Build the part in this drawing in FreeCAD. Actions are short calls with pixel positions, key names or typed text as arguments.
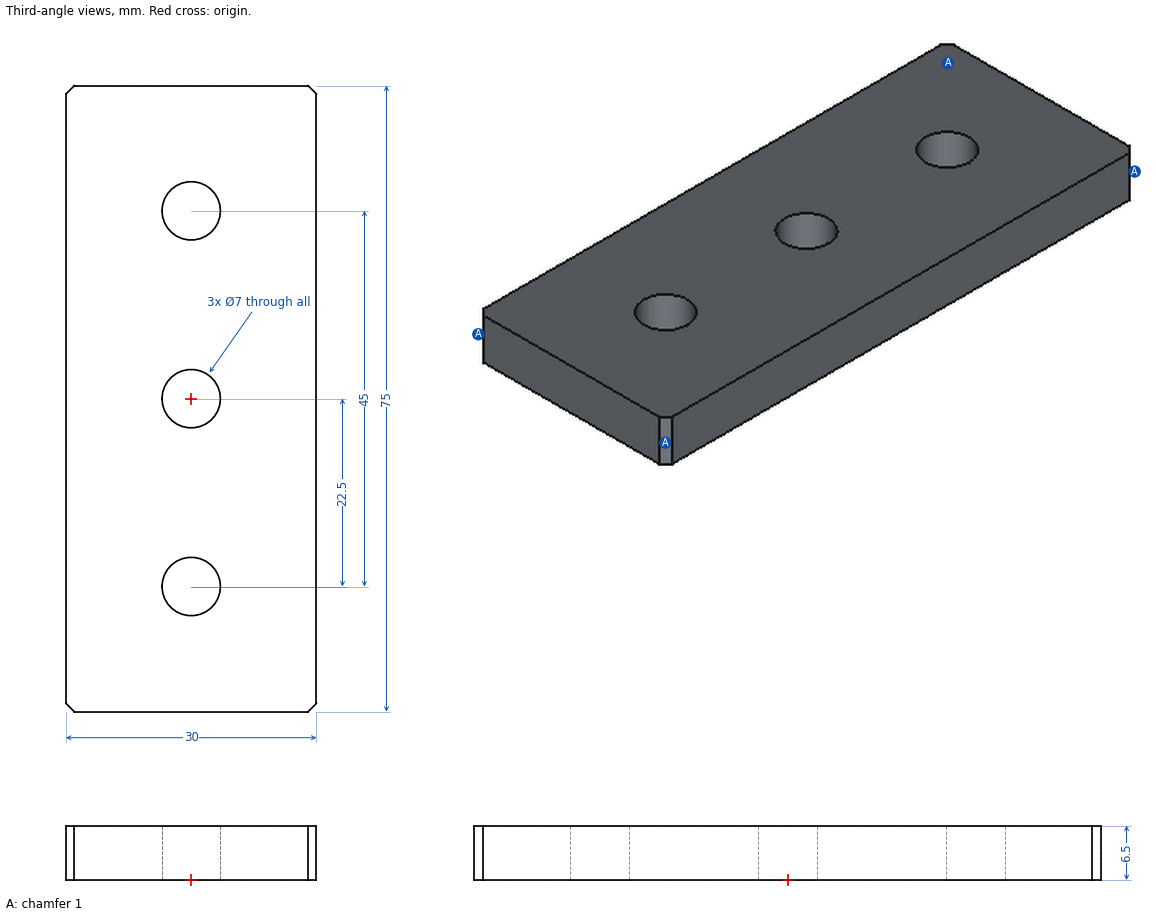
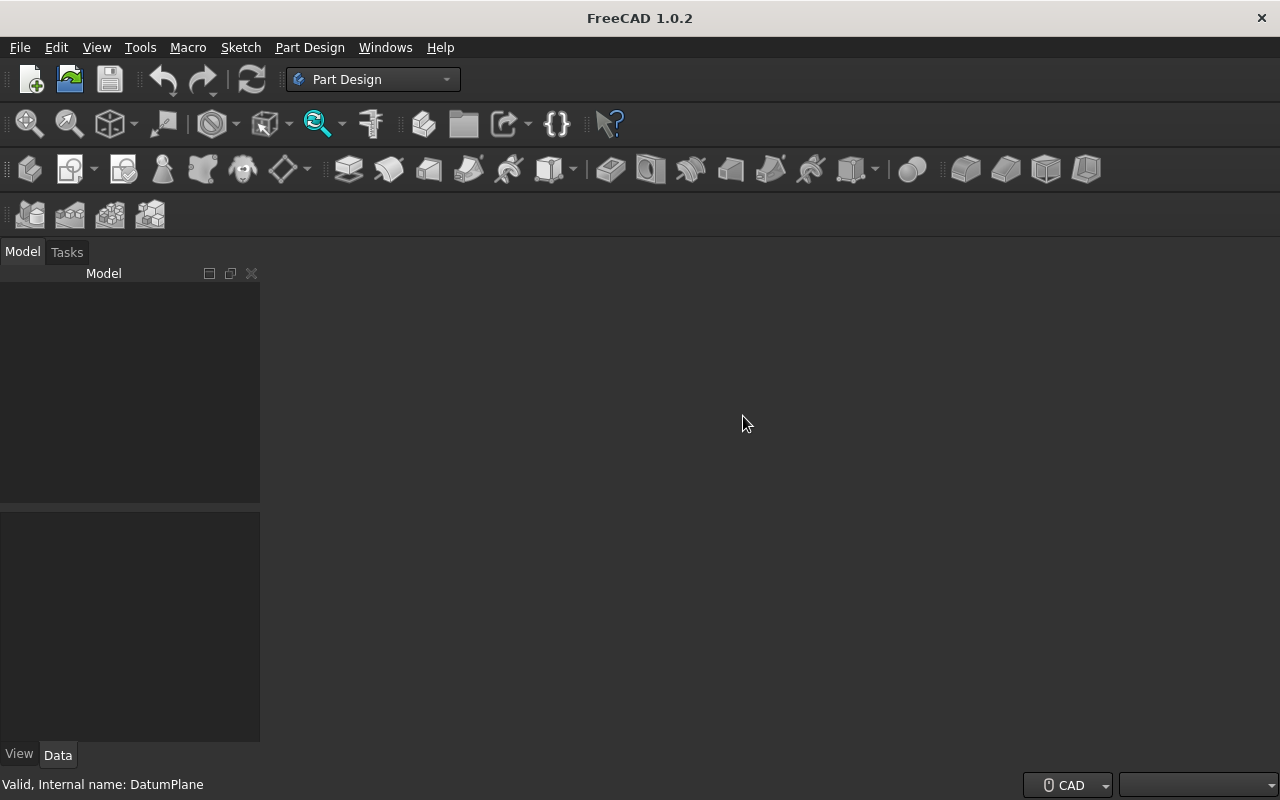
key(ctrl+n)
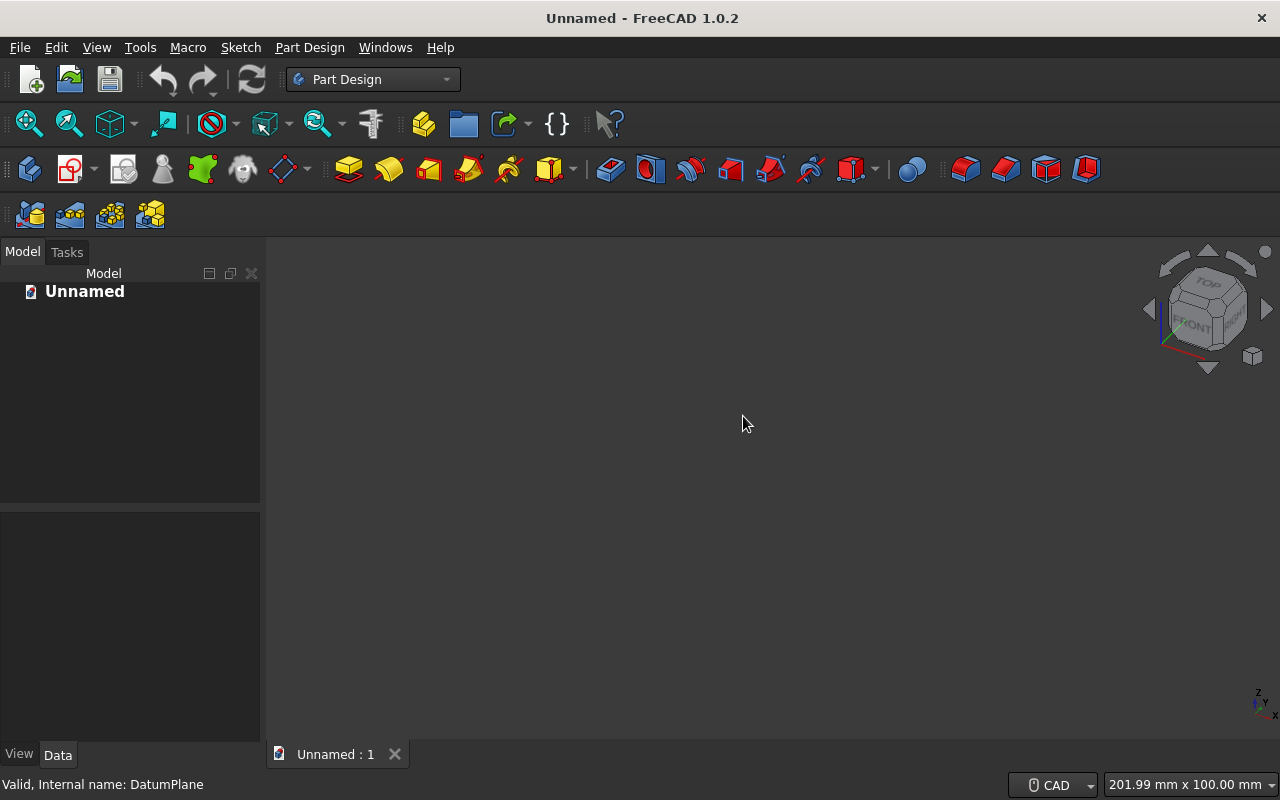
click(70, 170)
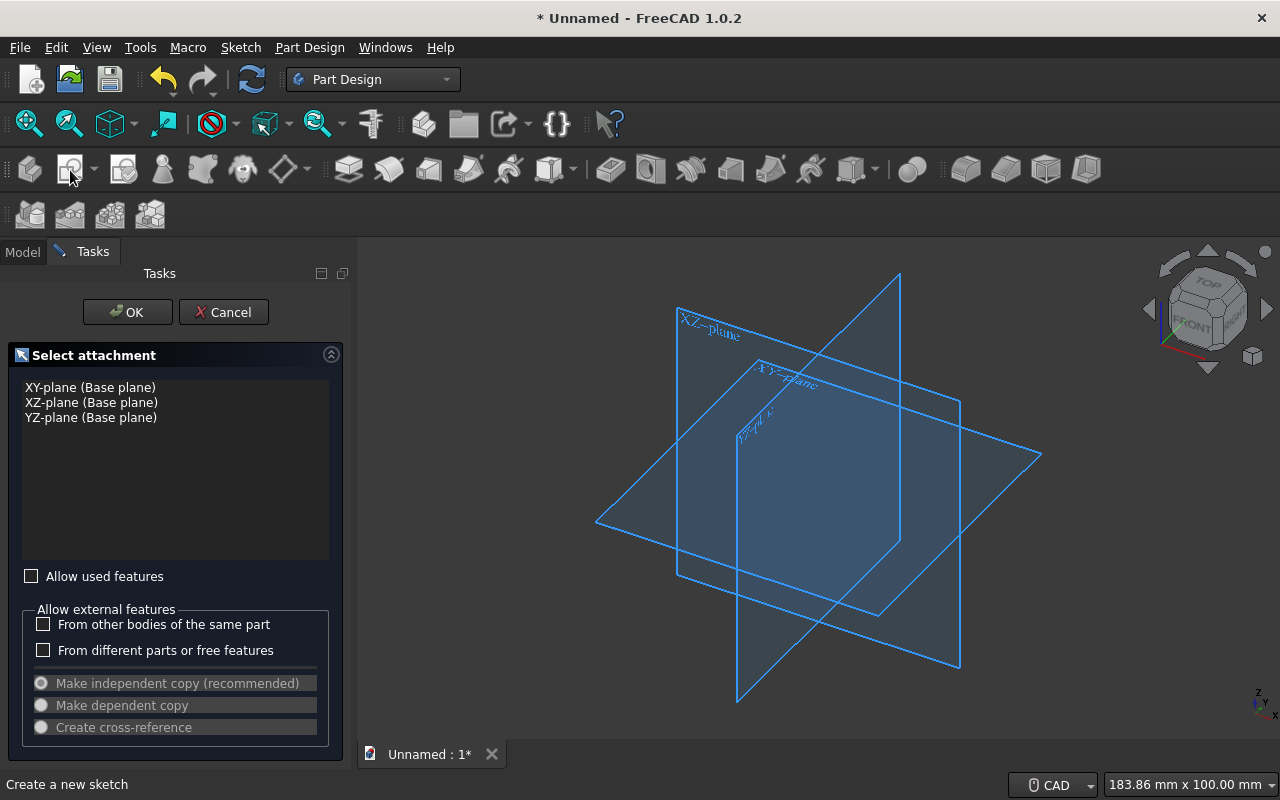
click(82, 388)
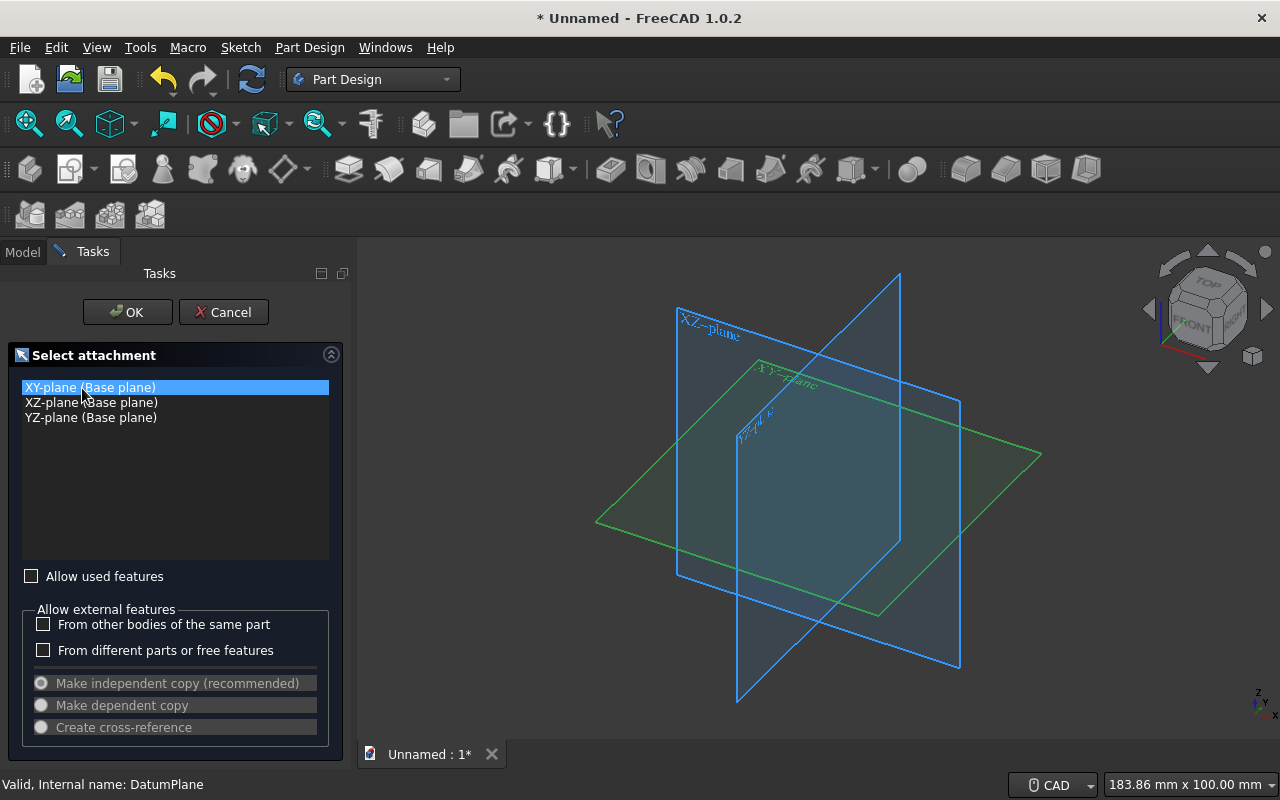
click(128, 312)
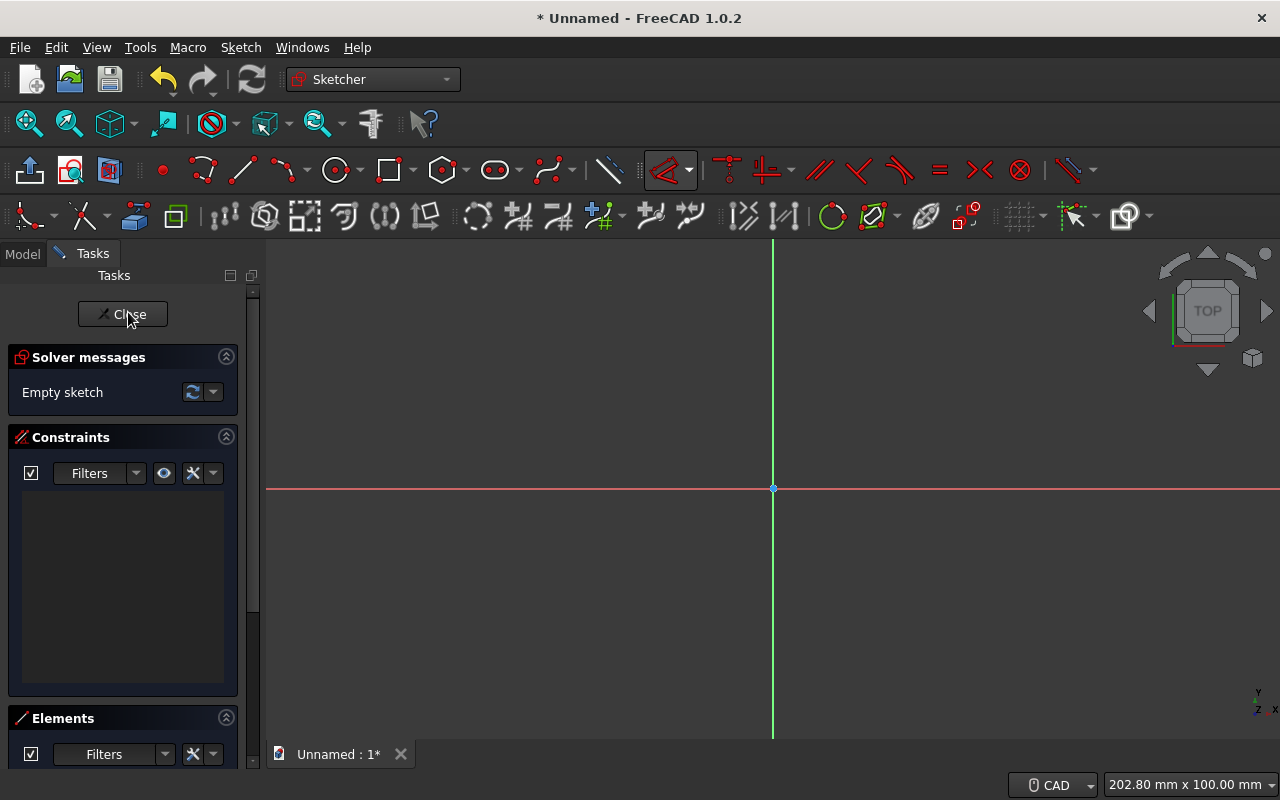
key(g)
key(v)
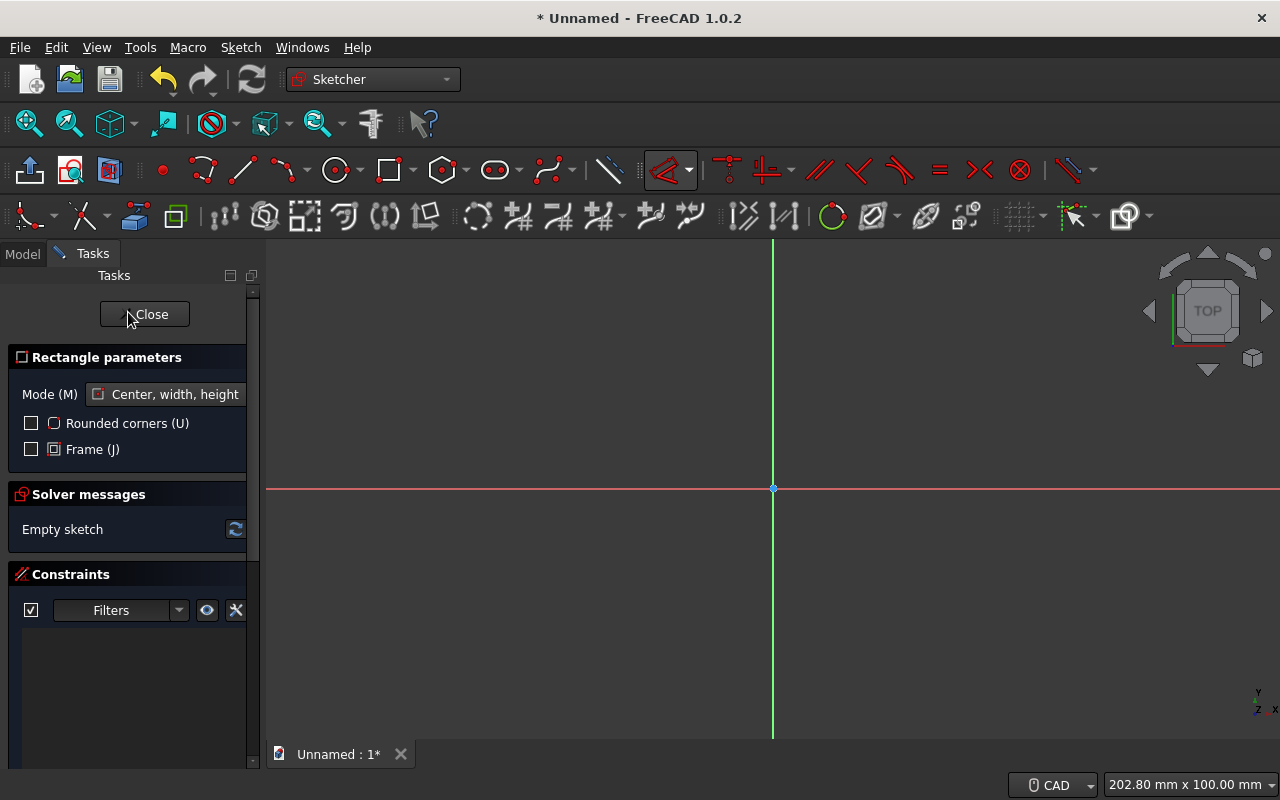
click(773, 489)
click(848, 302)
key(Escape)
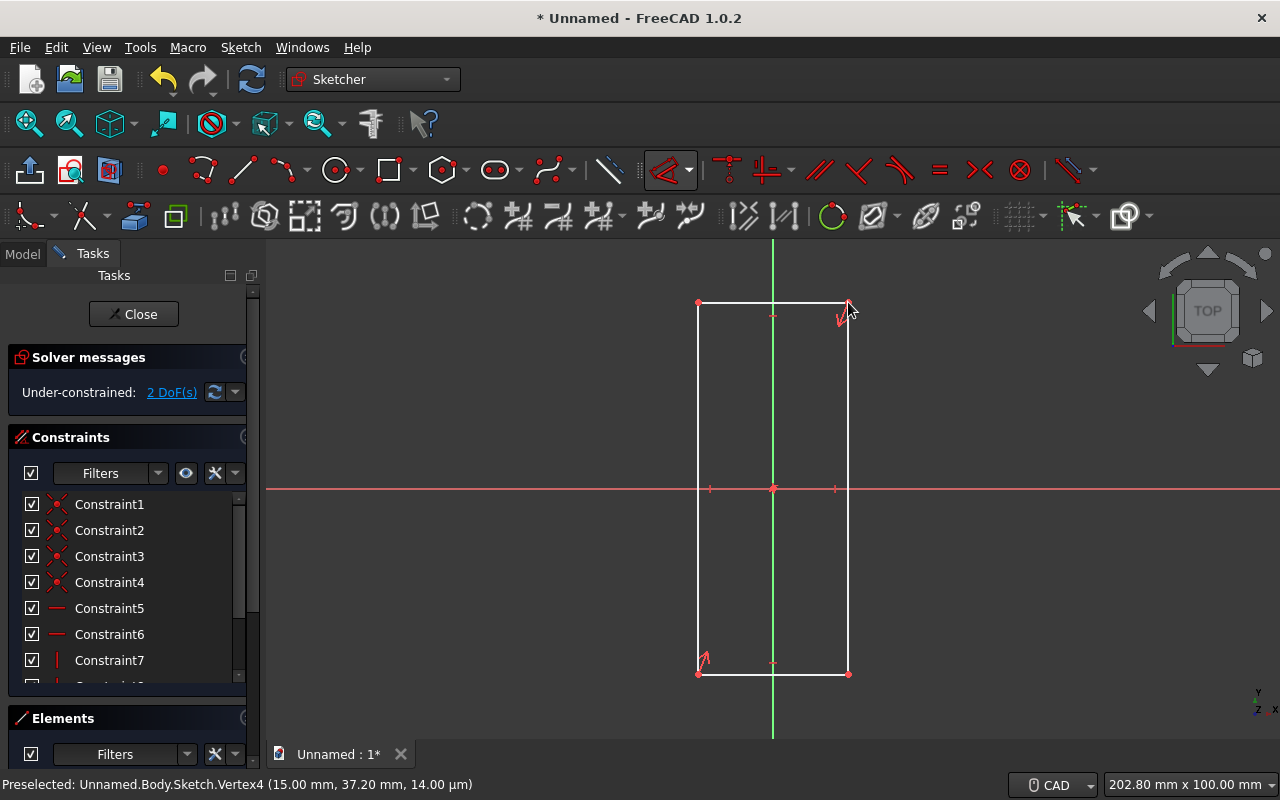
key(d)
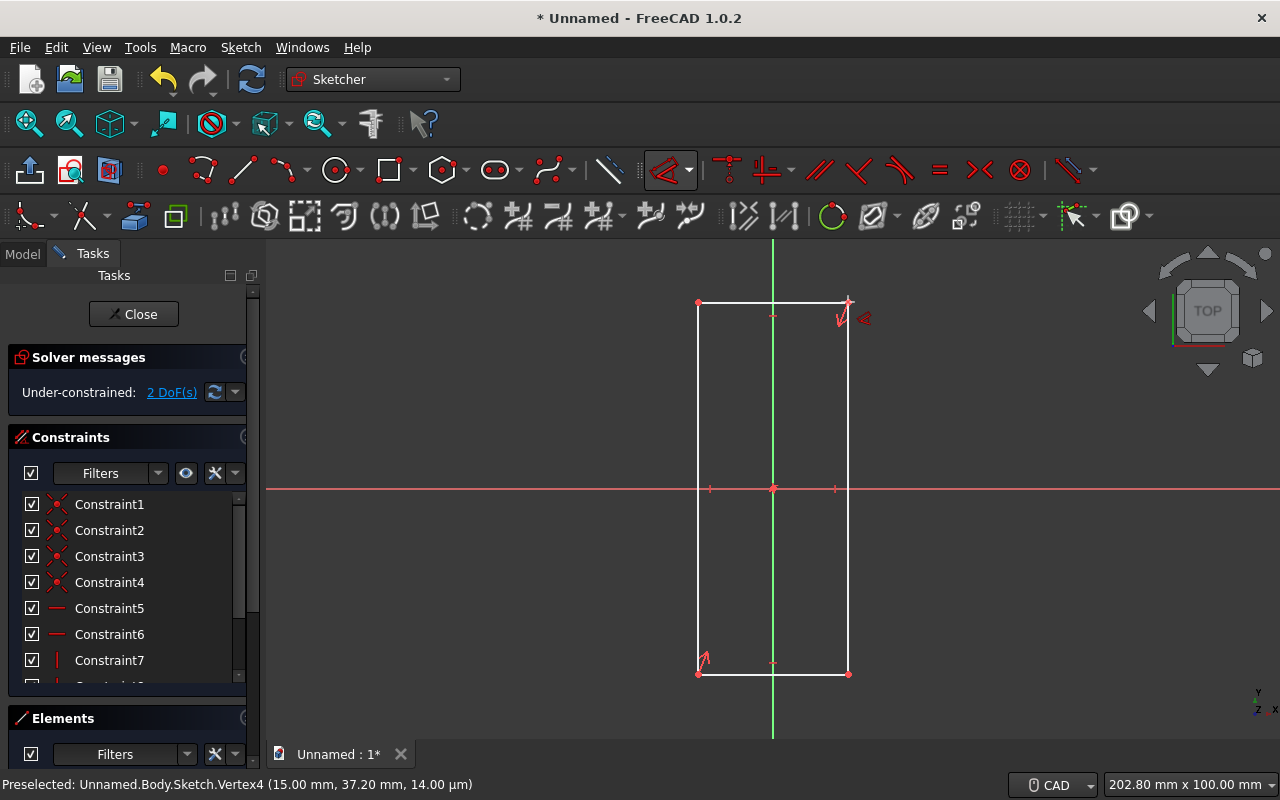
click(743, 675)
click(739, 709)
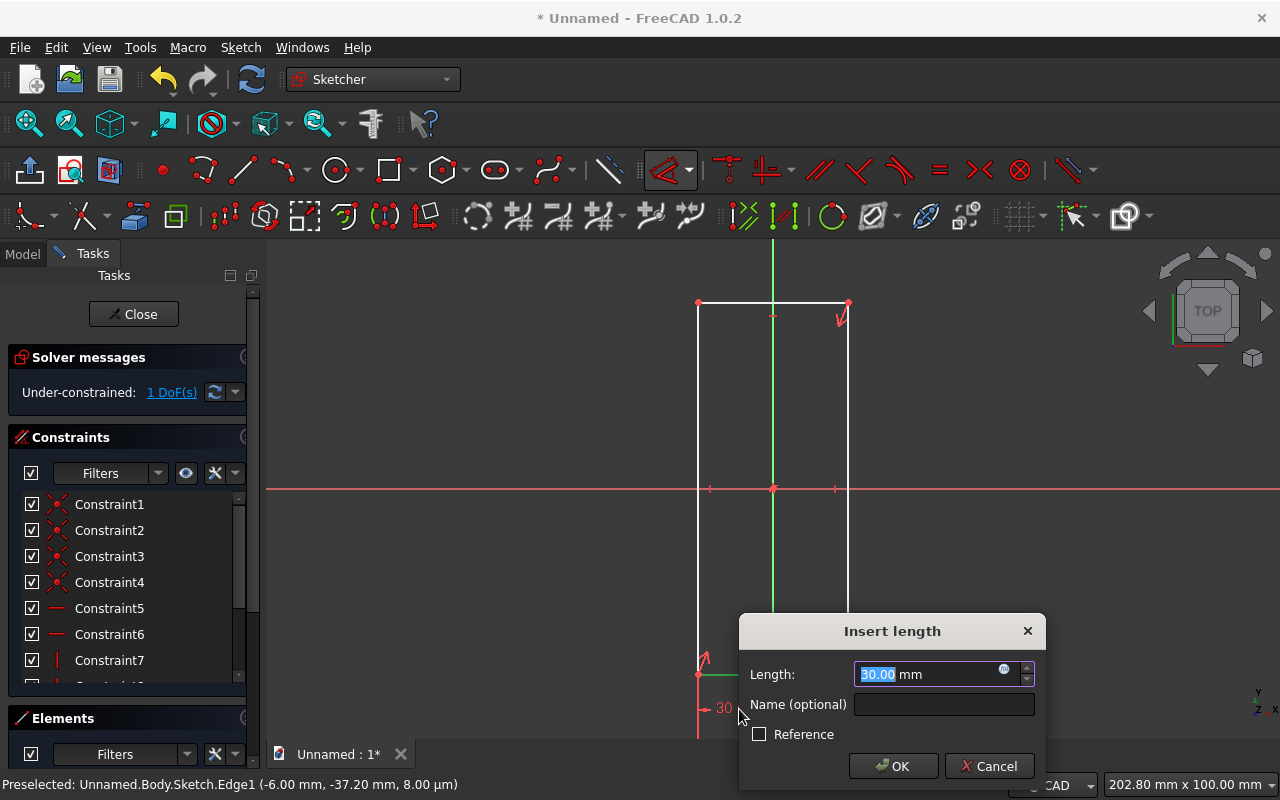
text(30)
key(Return)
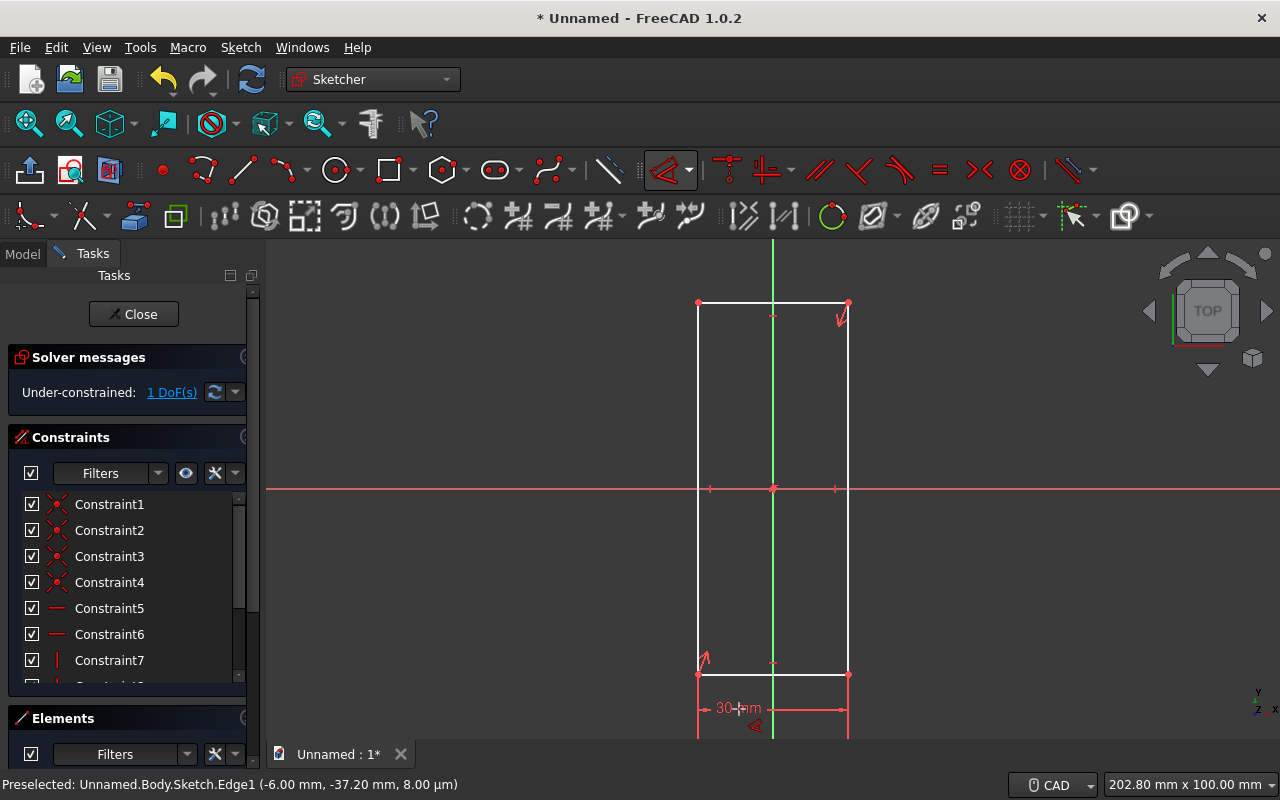
click(848, 563)
click(882, 403)